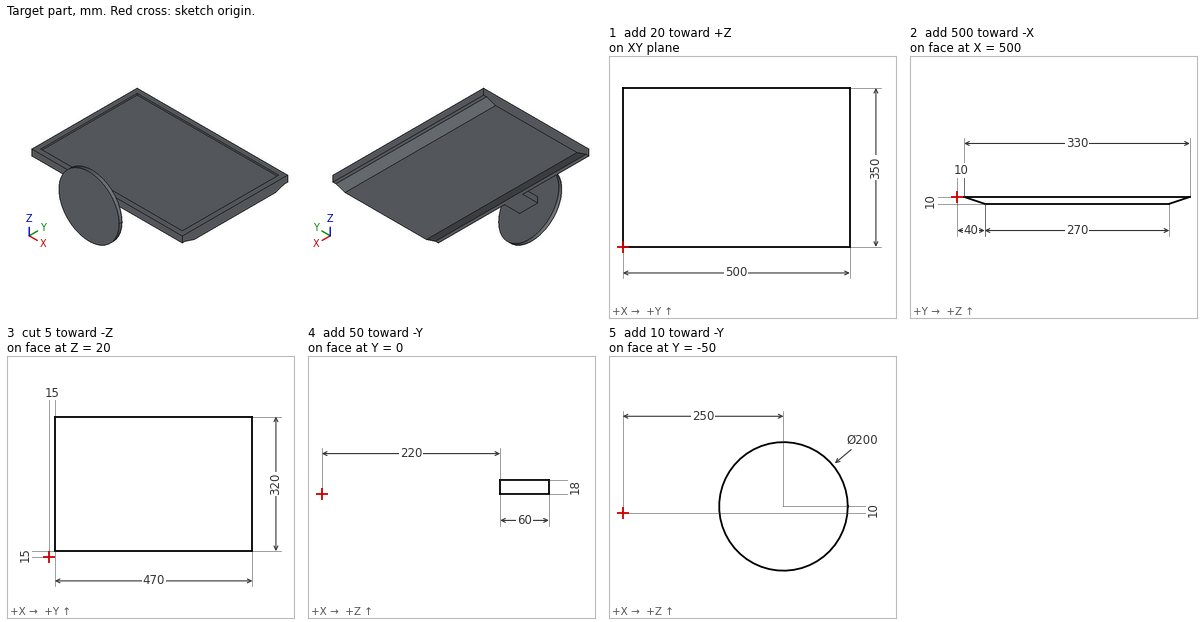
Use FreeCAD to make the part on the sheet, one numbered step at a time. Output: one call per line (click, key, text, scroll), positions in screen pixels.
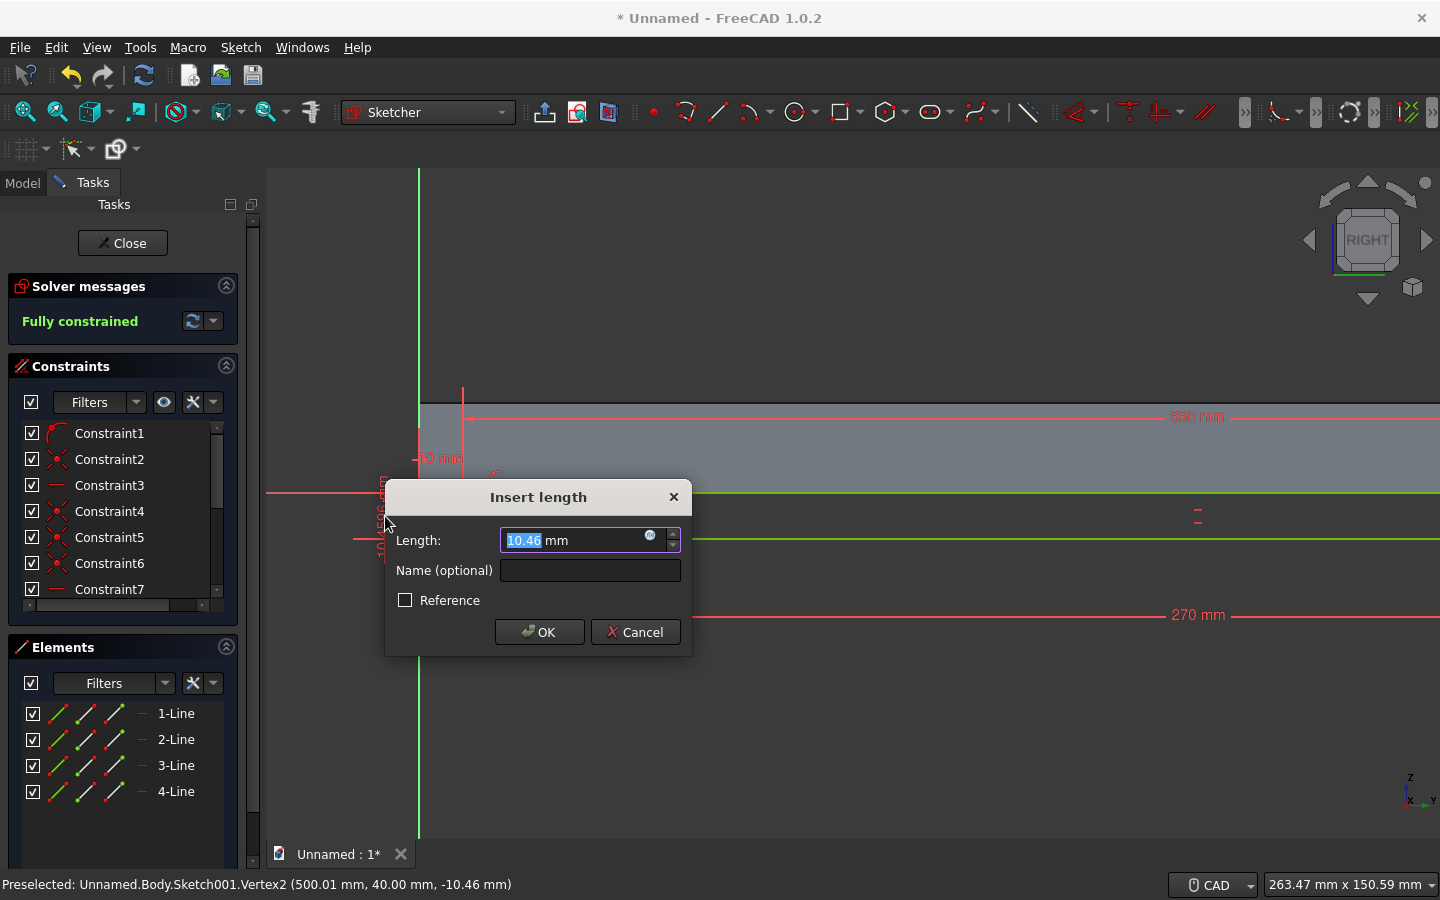
text(10)
key(Return)
key(Escape)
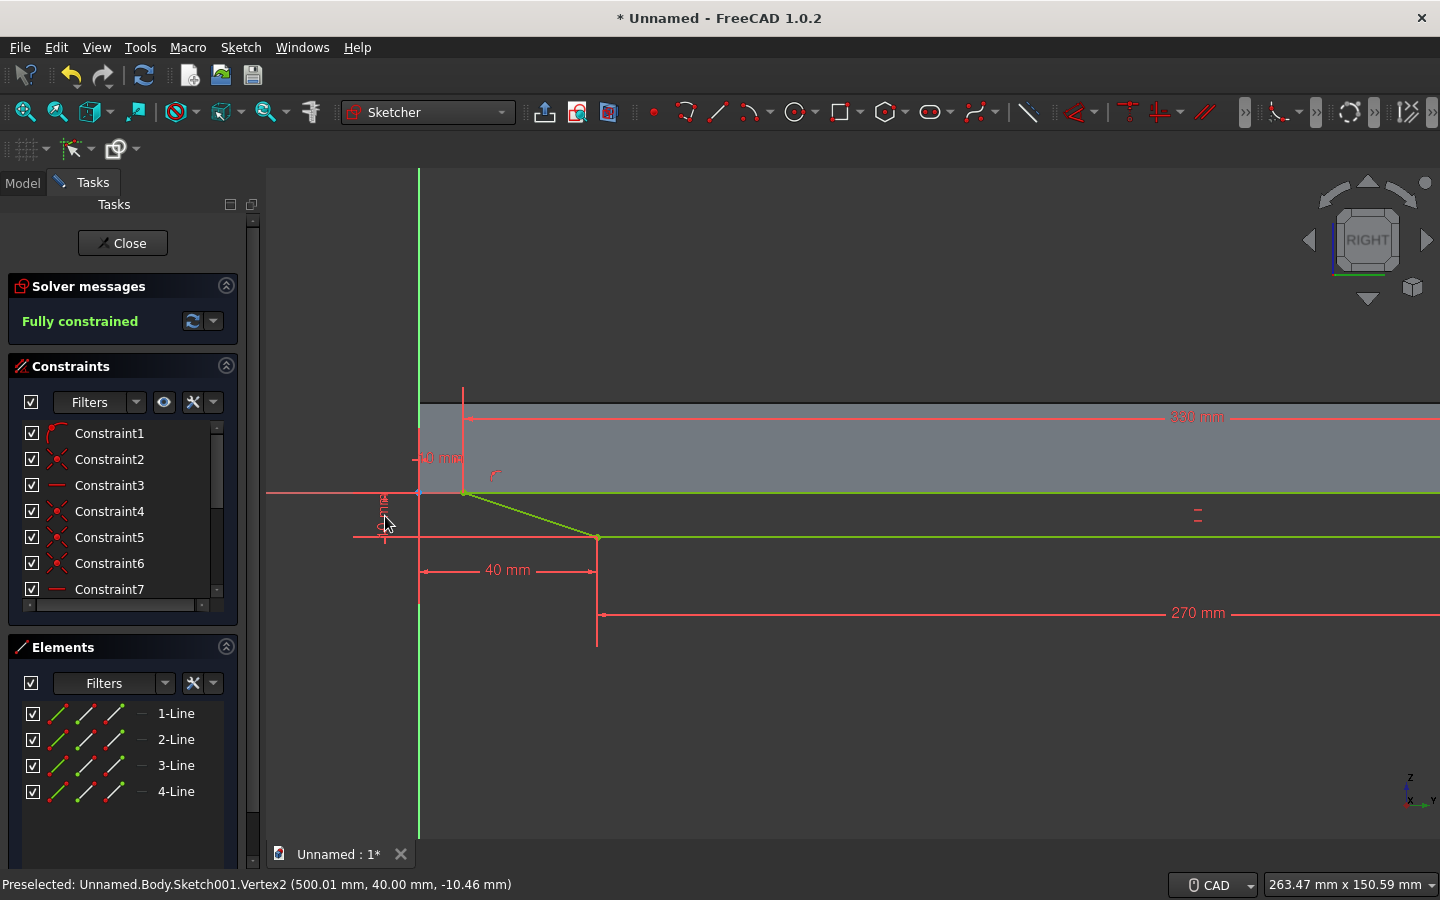
click(123, 243)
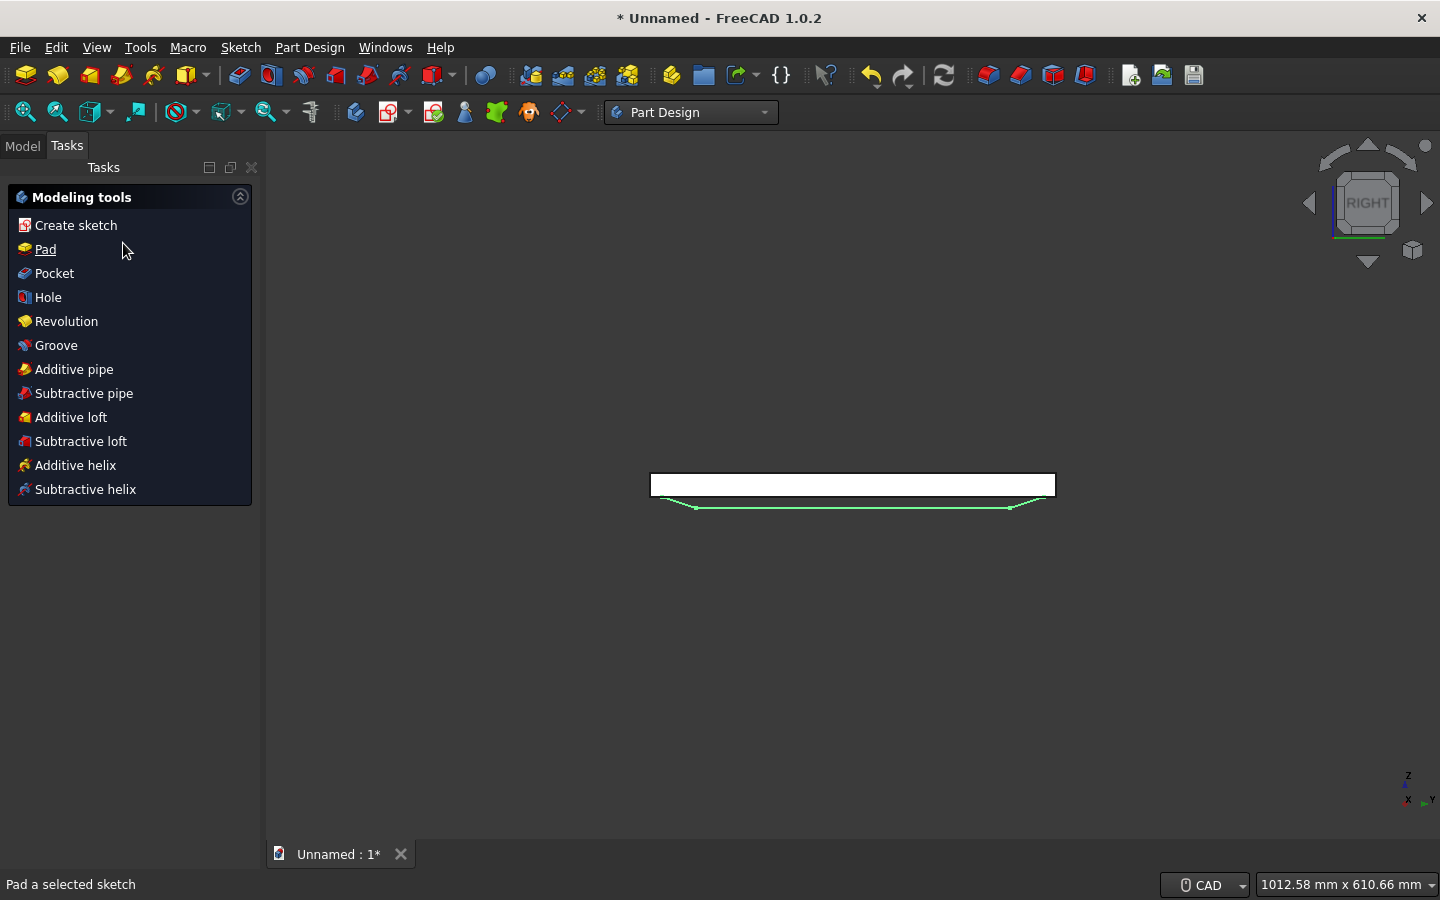
click(26, 76)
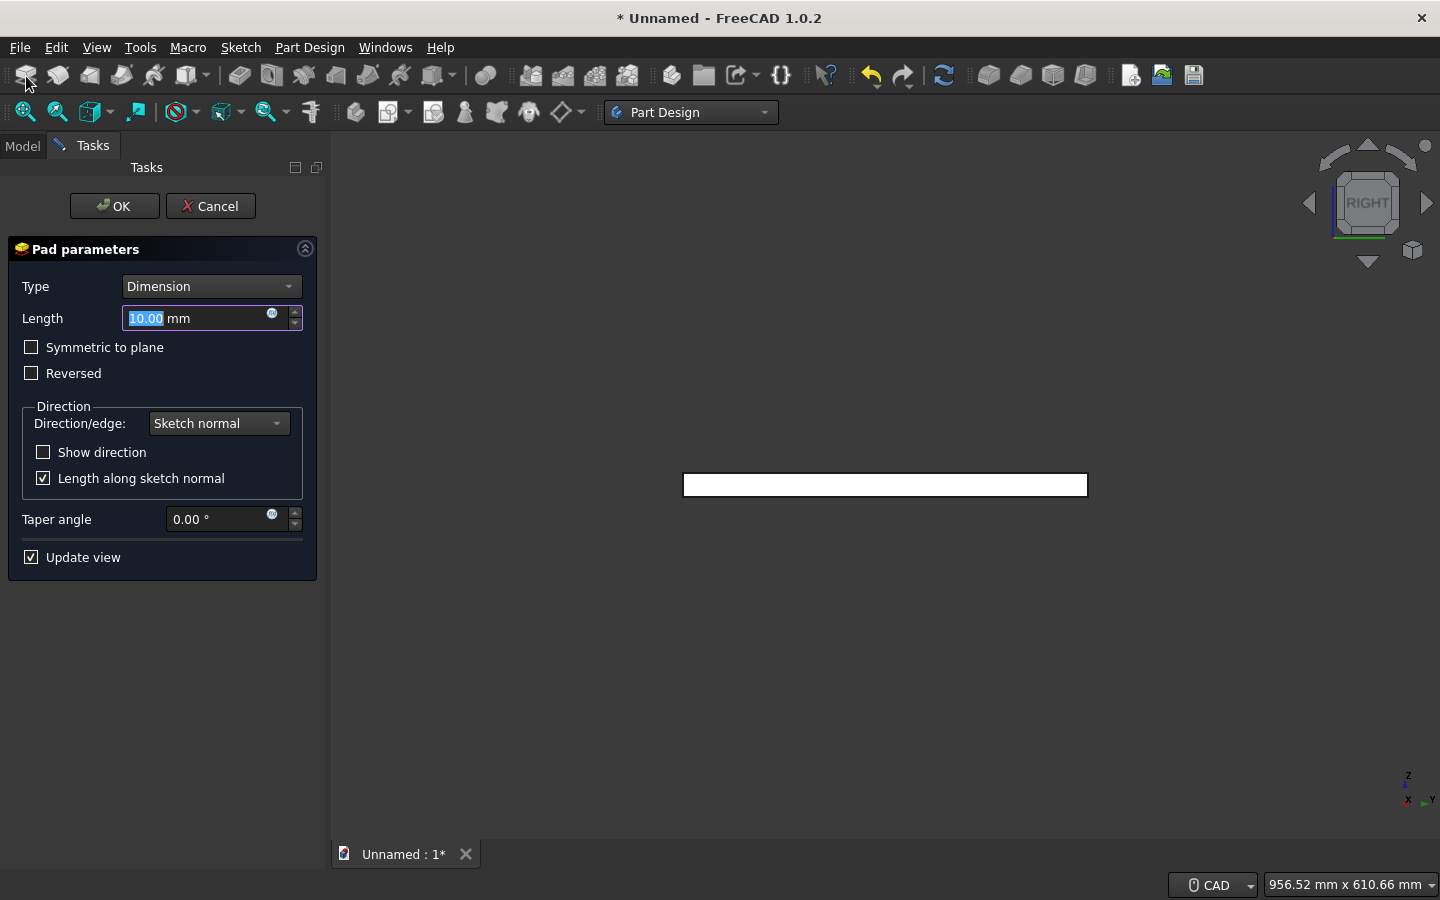
text(500)
key(Tab)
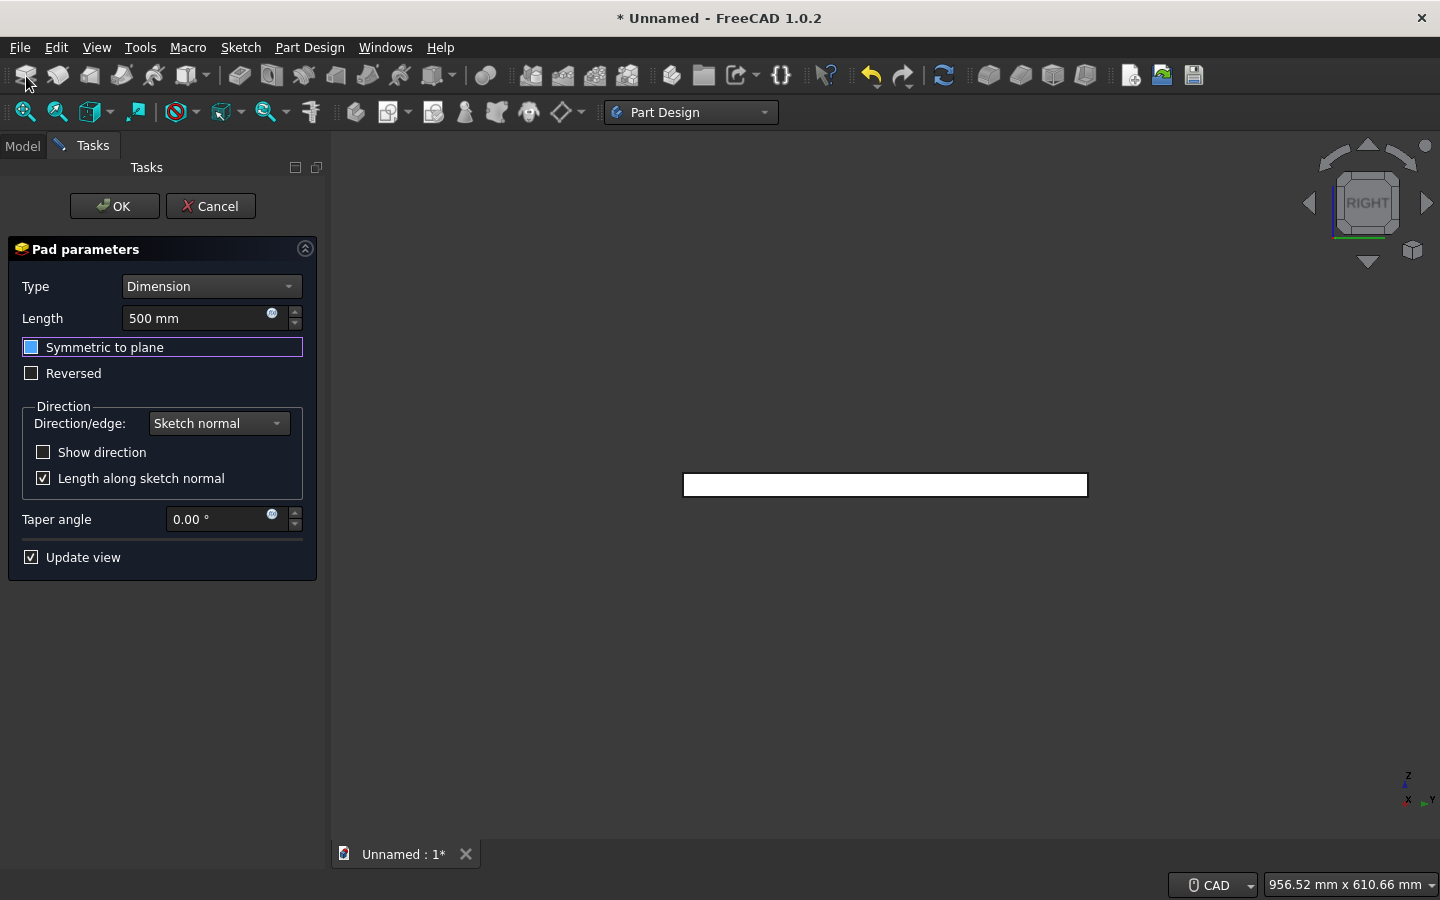
click(30, 373)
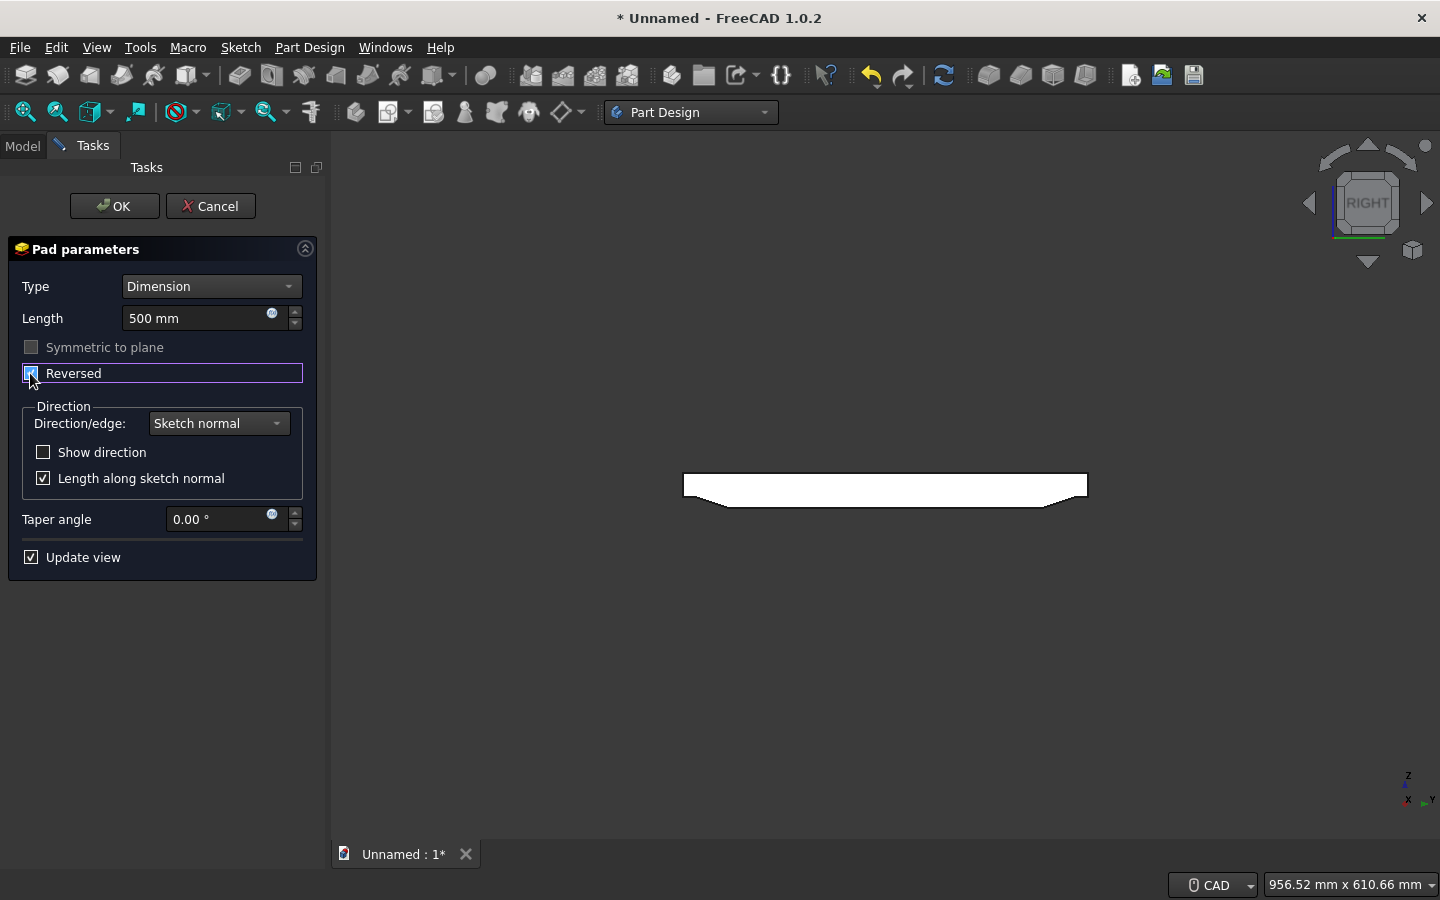
click(115, 206)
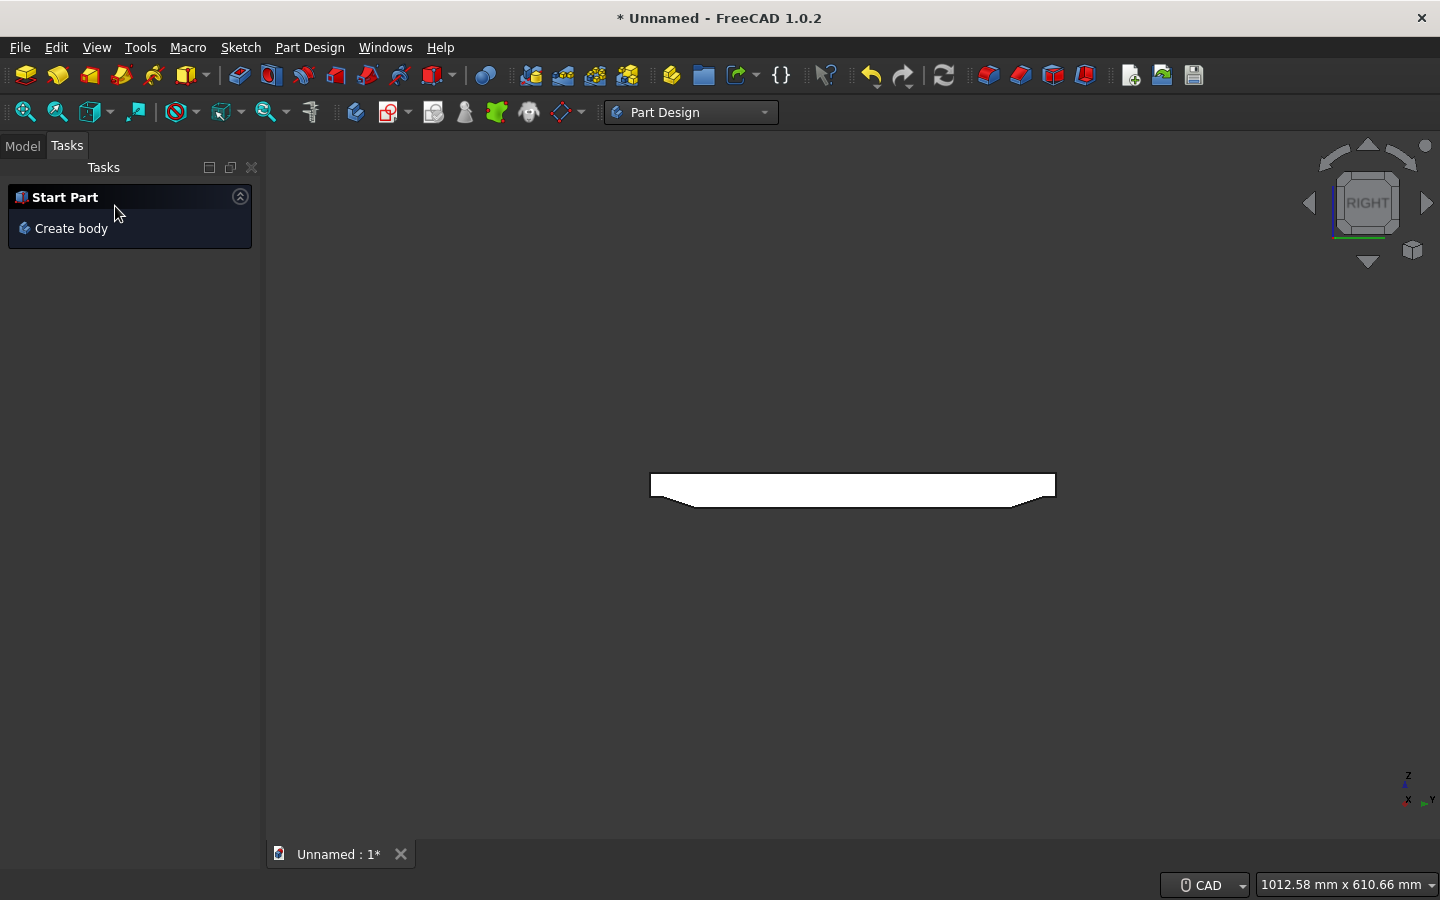
key(v)
key(f)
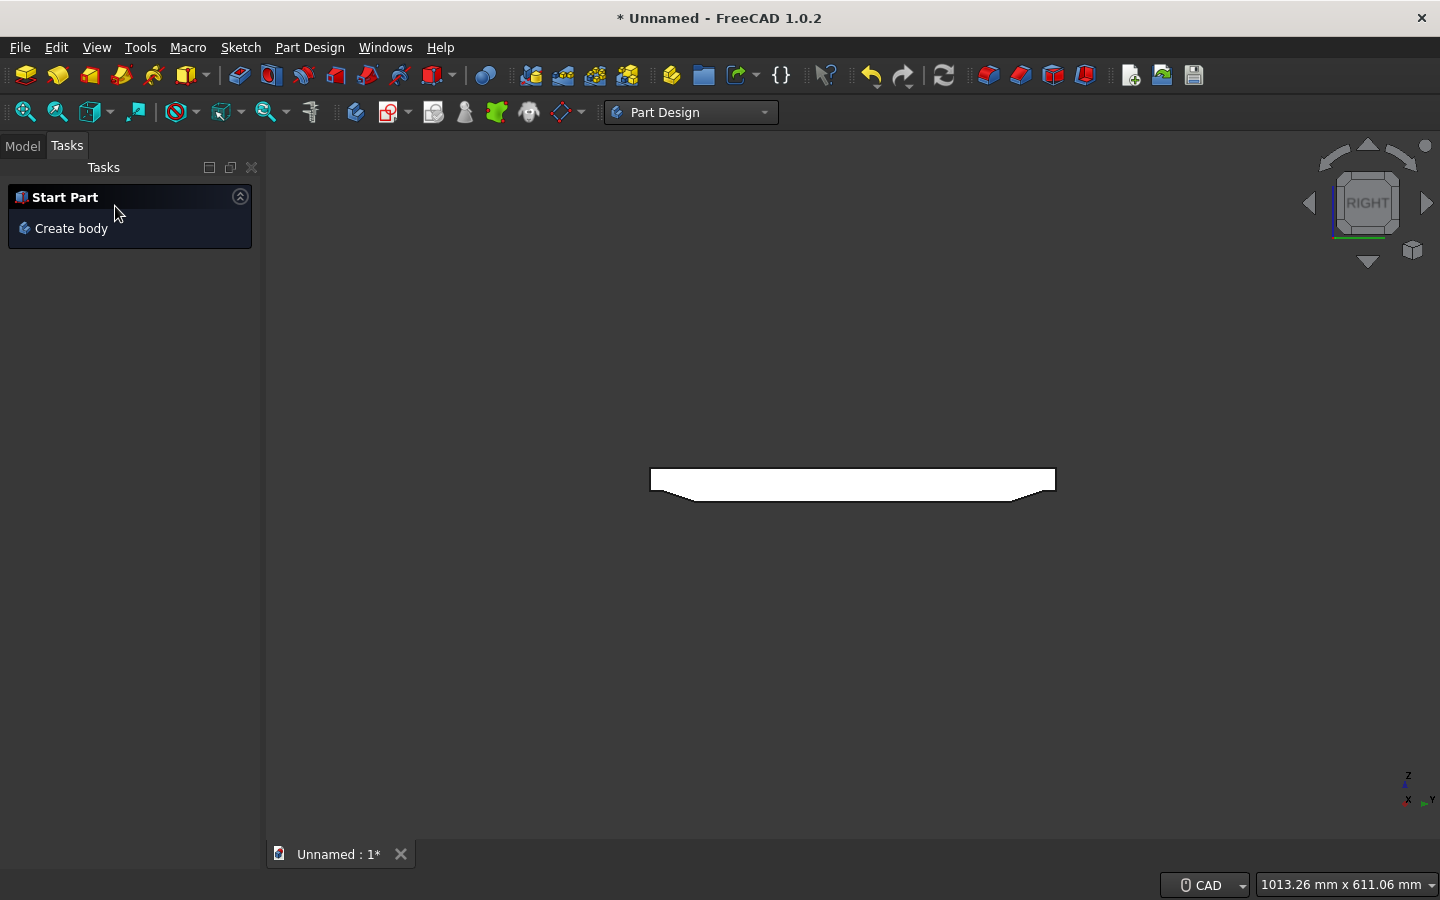
key(0)